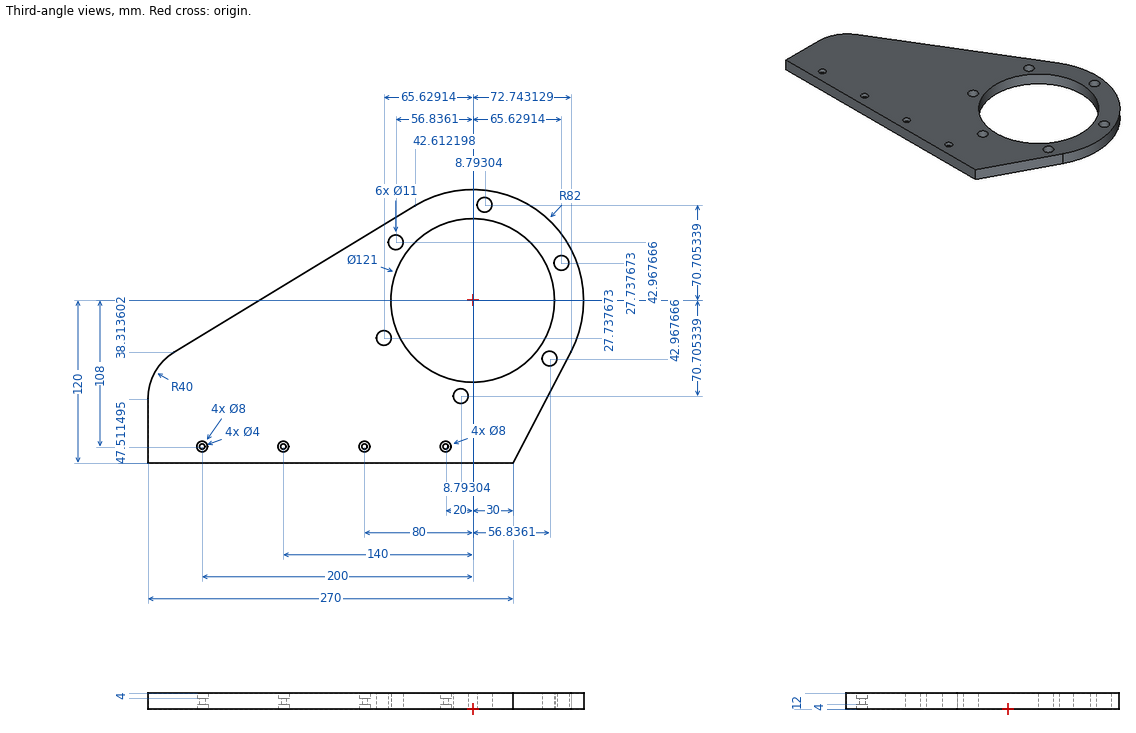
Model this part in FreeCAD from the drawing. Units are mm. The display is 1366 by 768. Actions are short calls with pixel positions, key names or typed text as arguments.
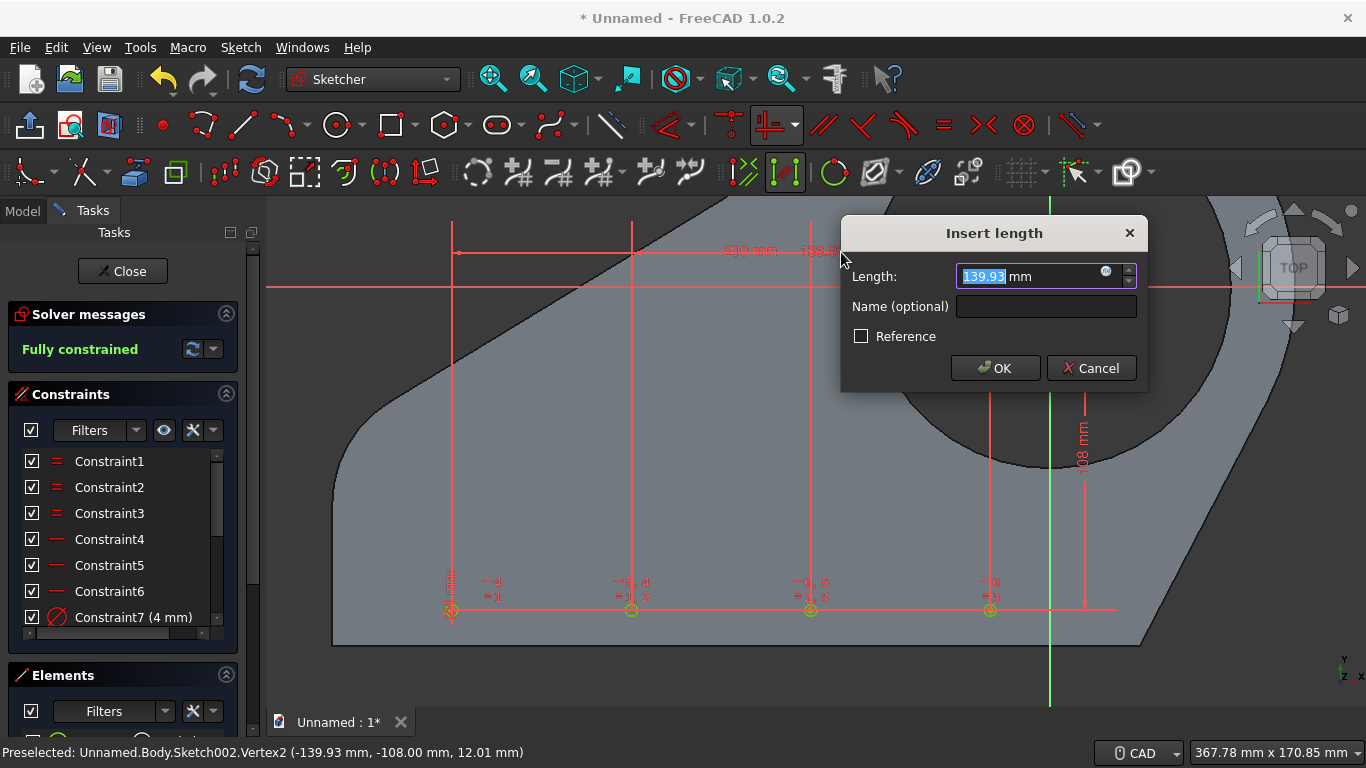
text(140)
key(Return)
key(Escape)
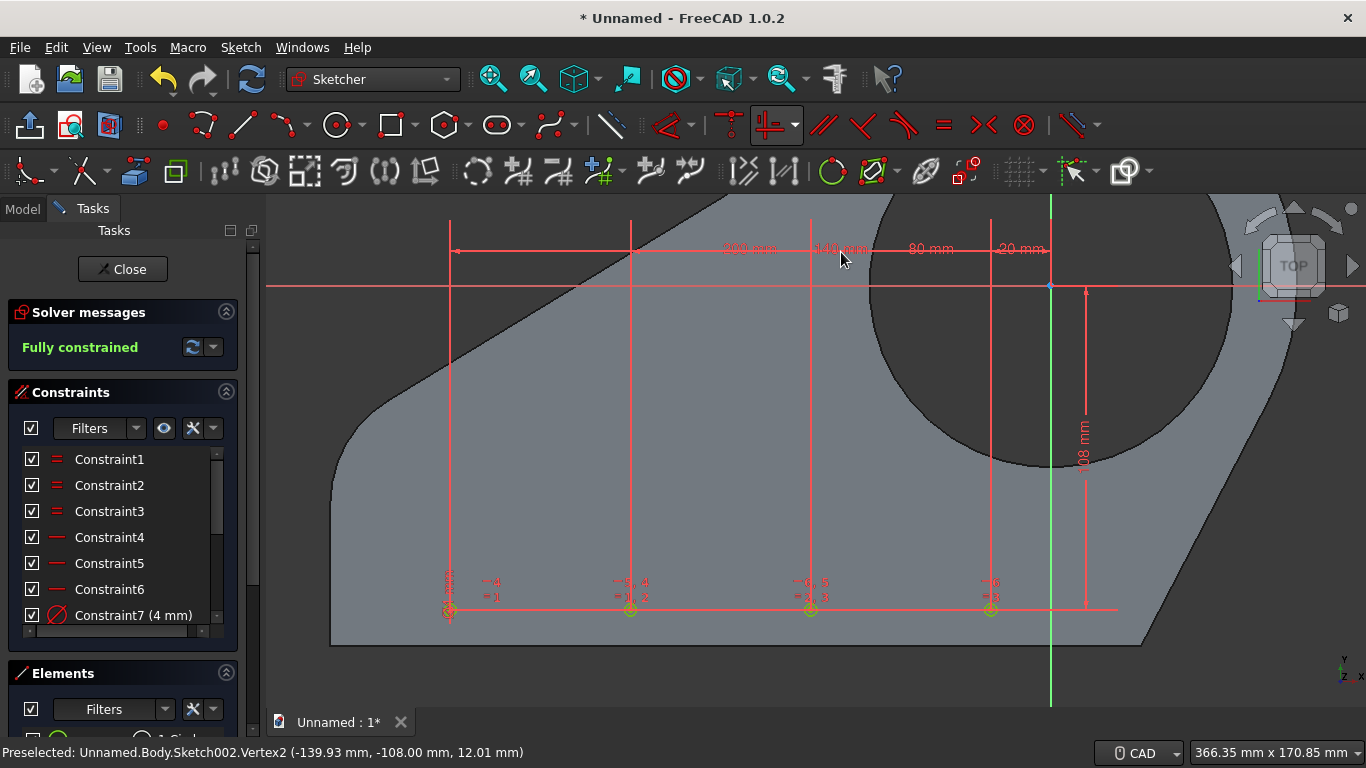
click(123, 269)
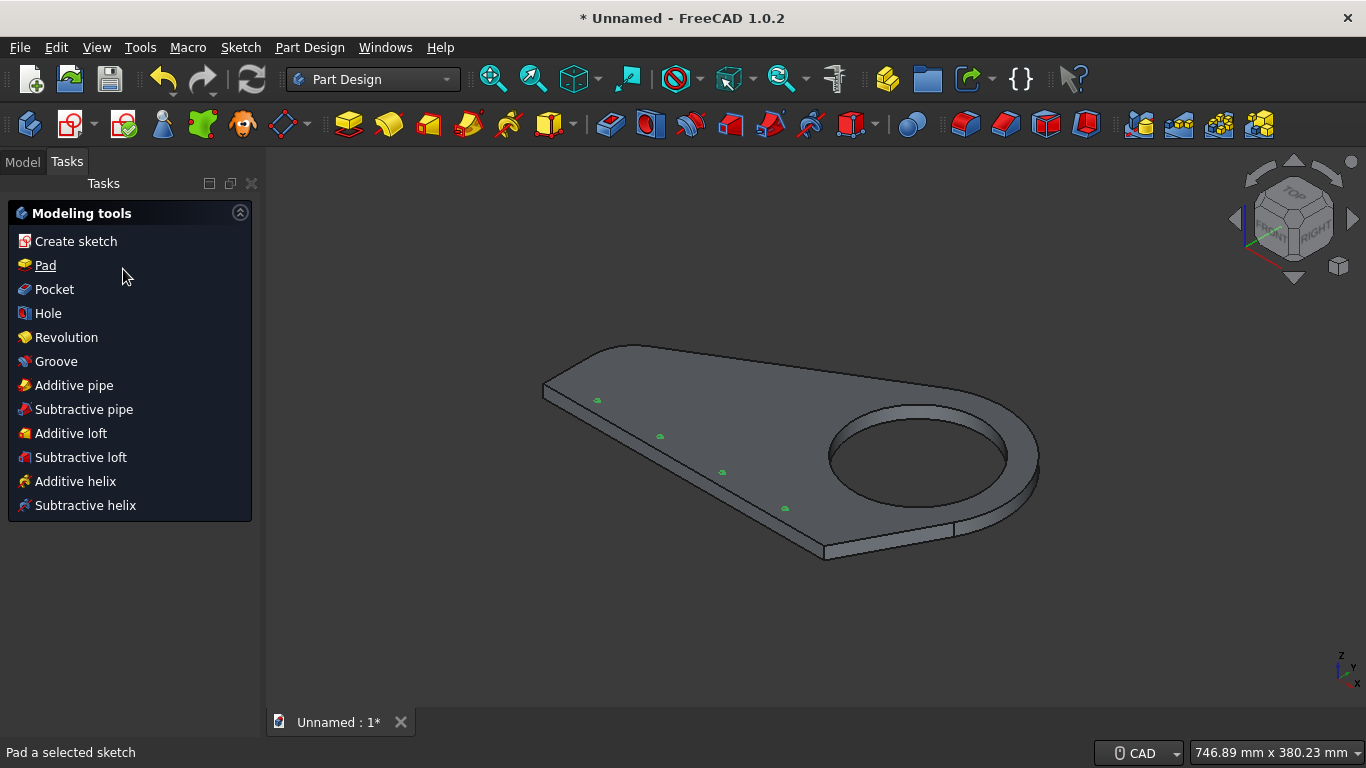
click(612, 124)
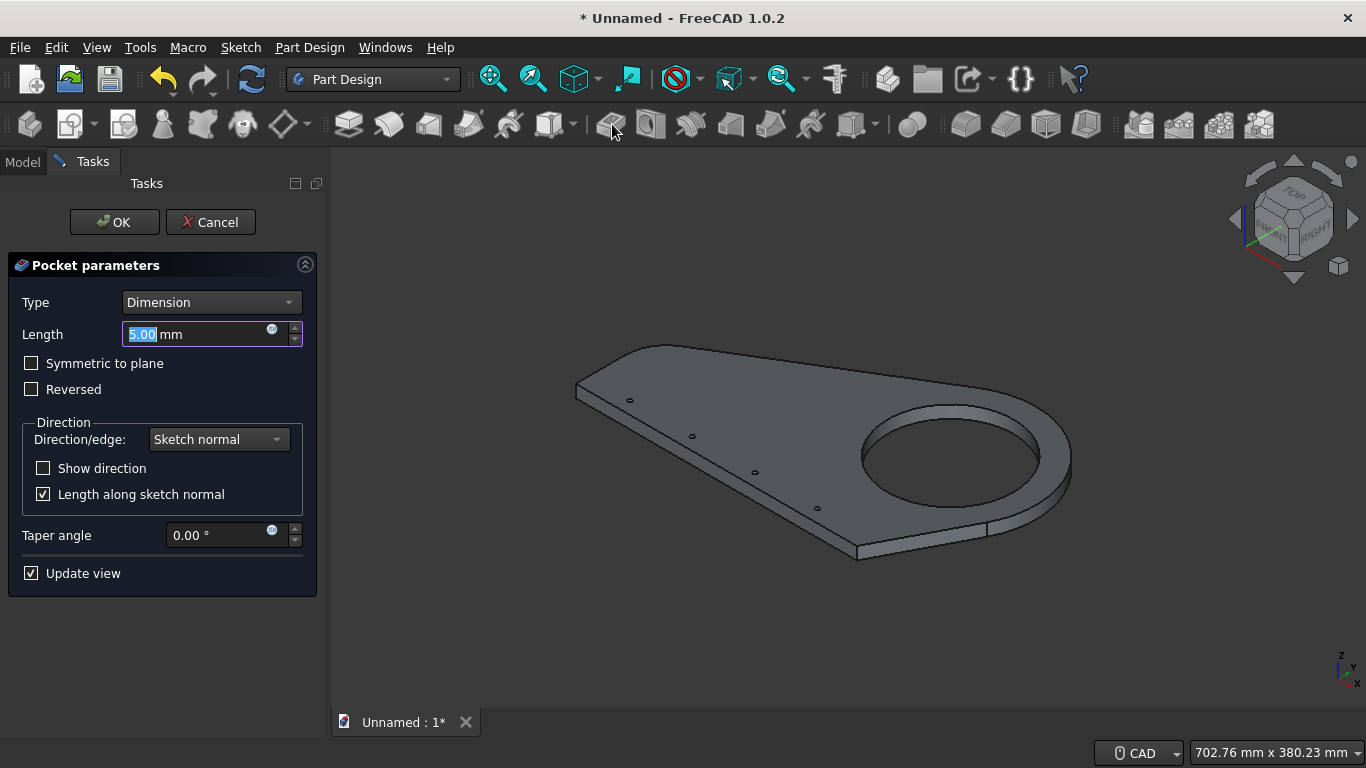
click(212, 302)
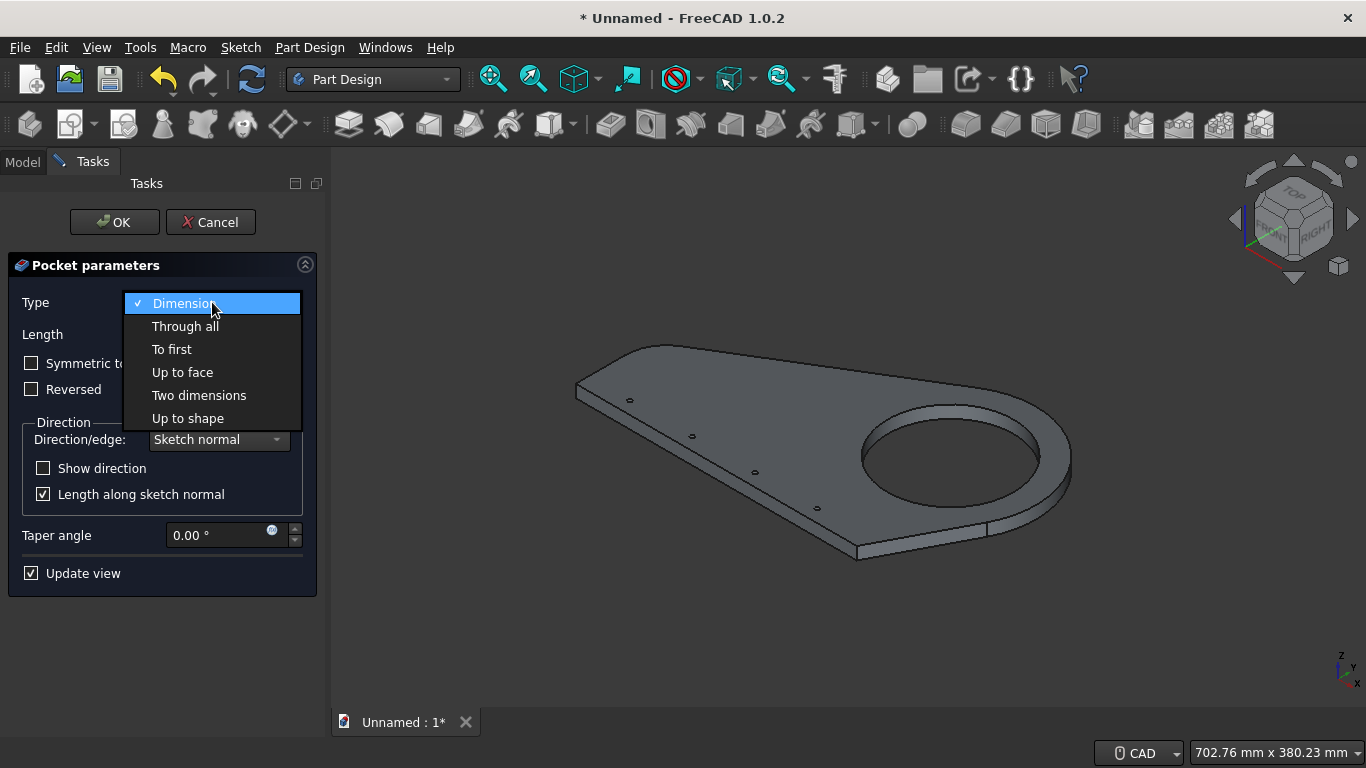
click(212, 326)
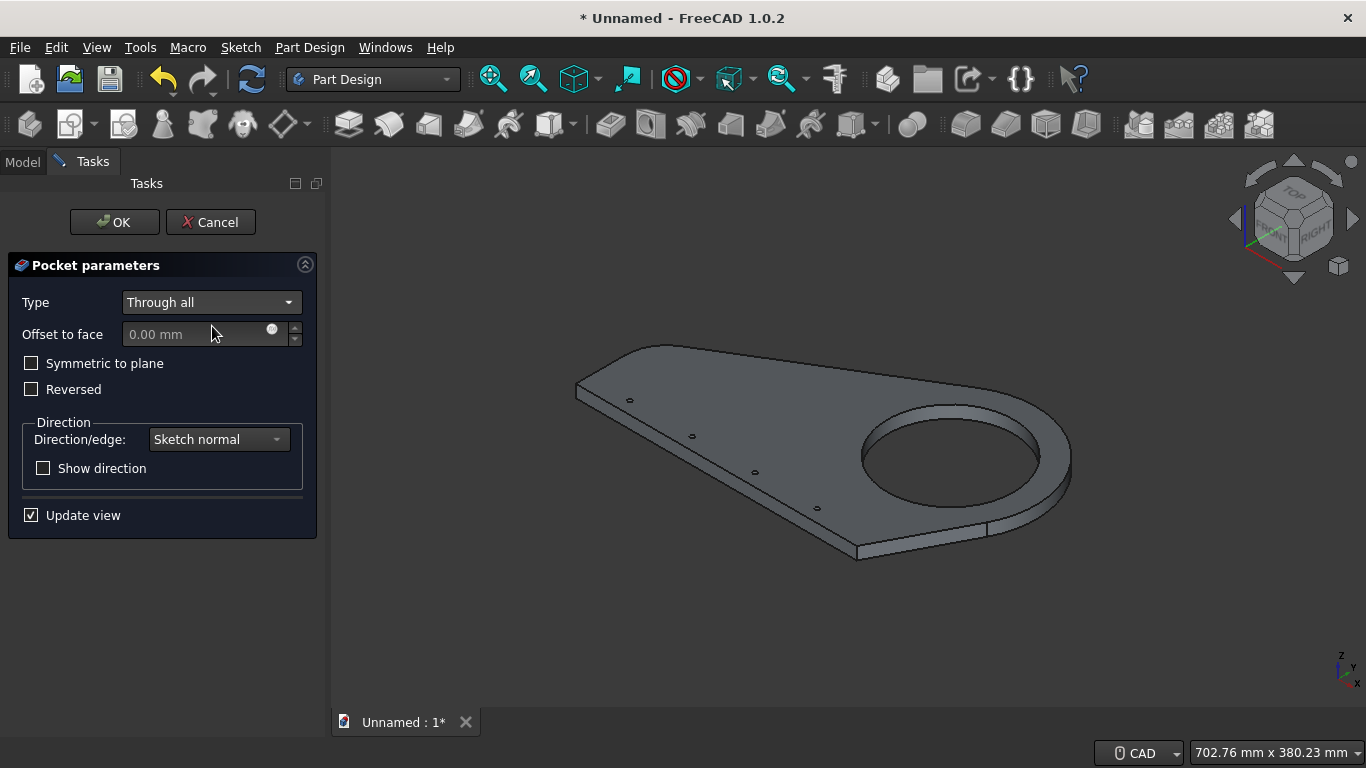
click(115, 222)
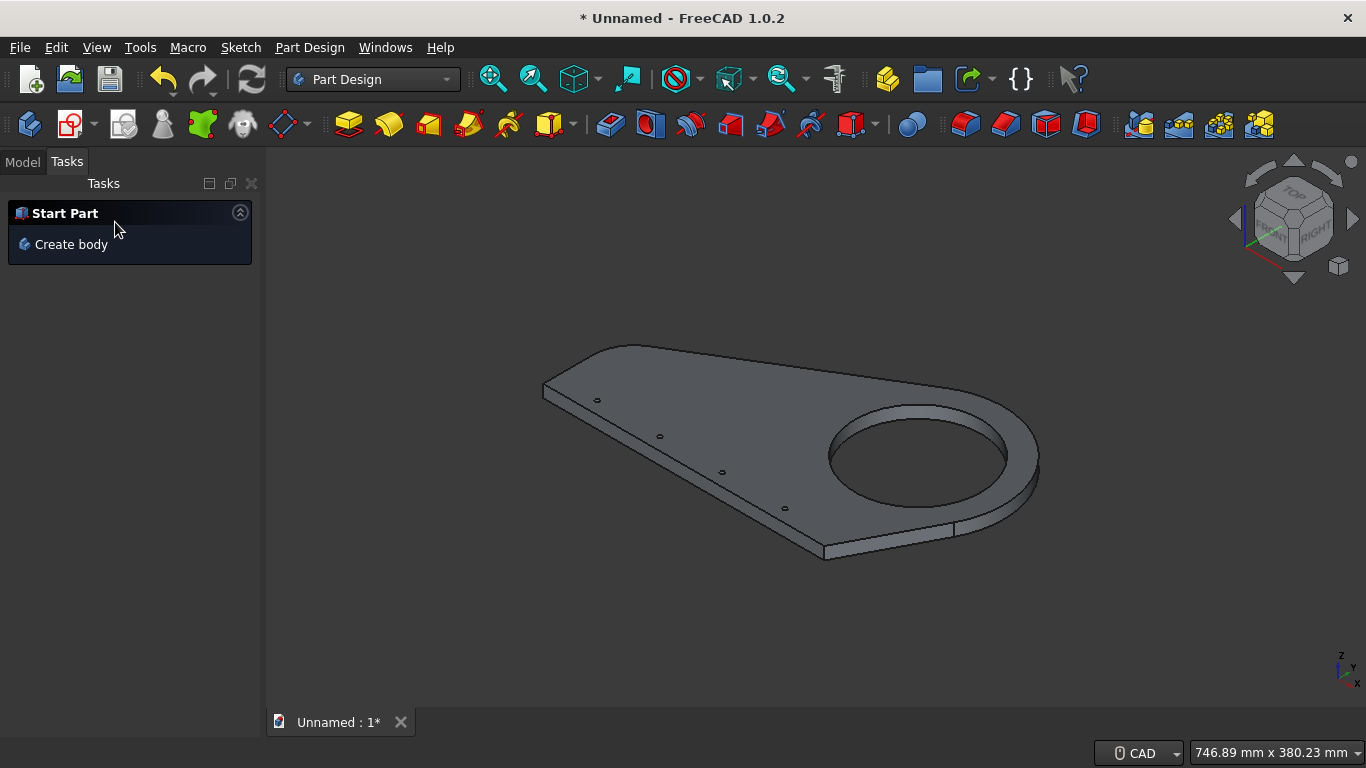
click(738, 408)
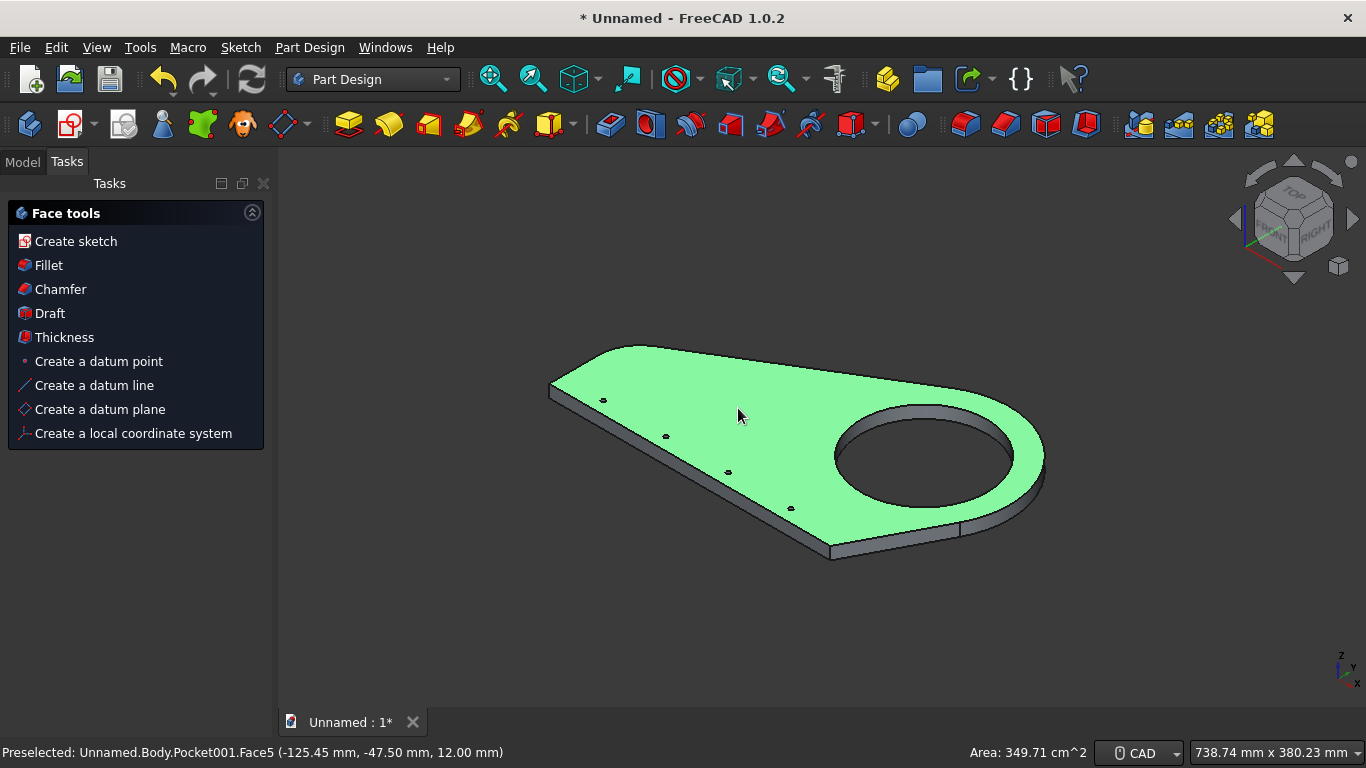
click(70, 124)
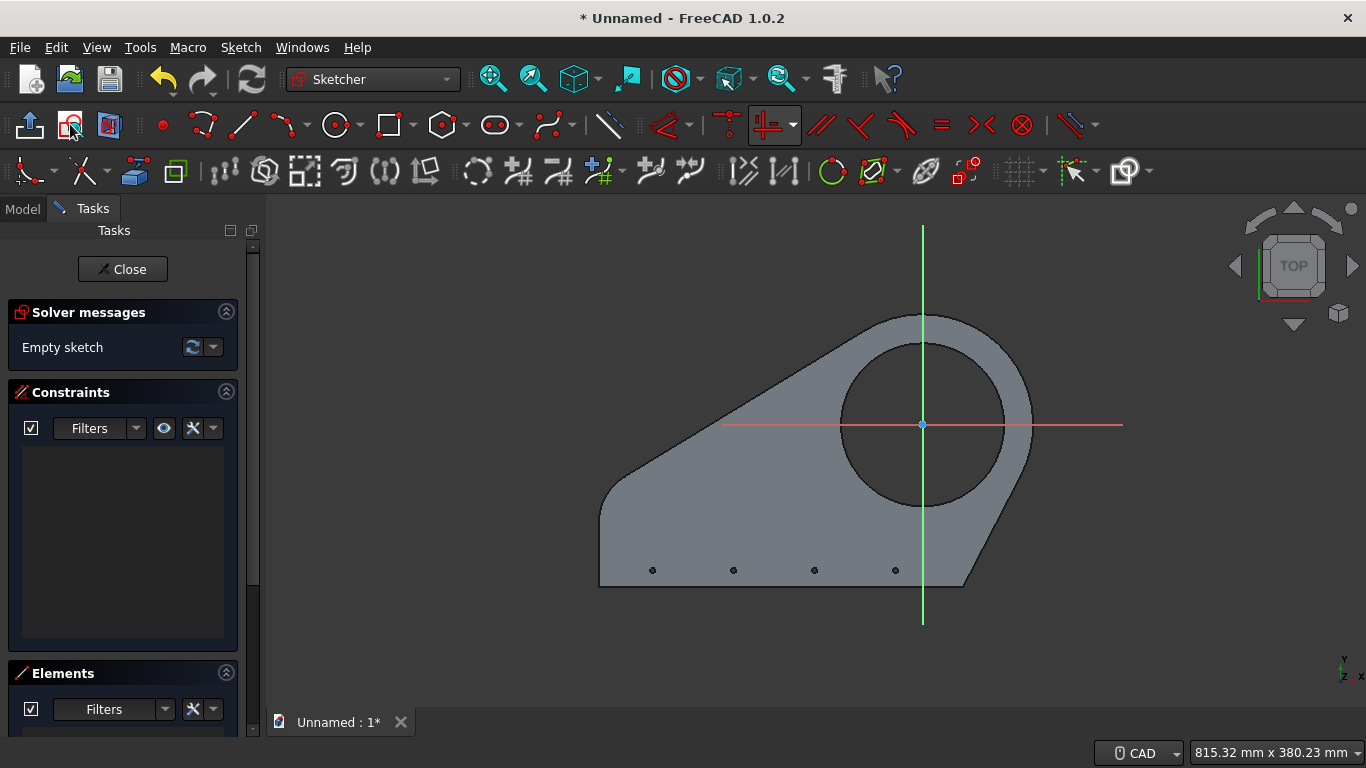
scroll(816, 541, up, 4)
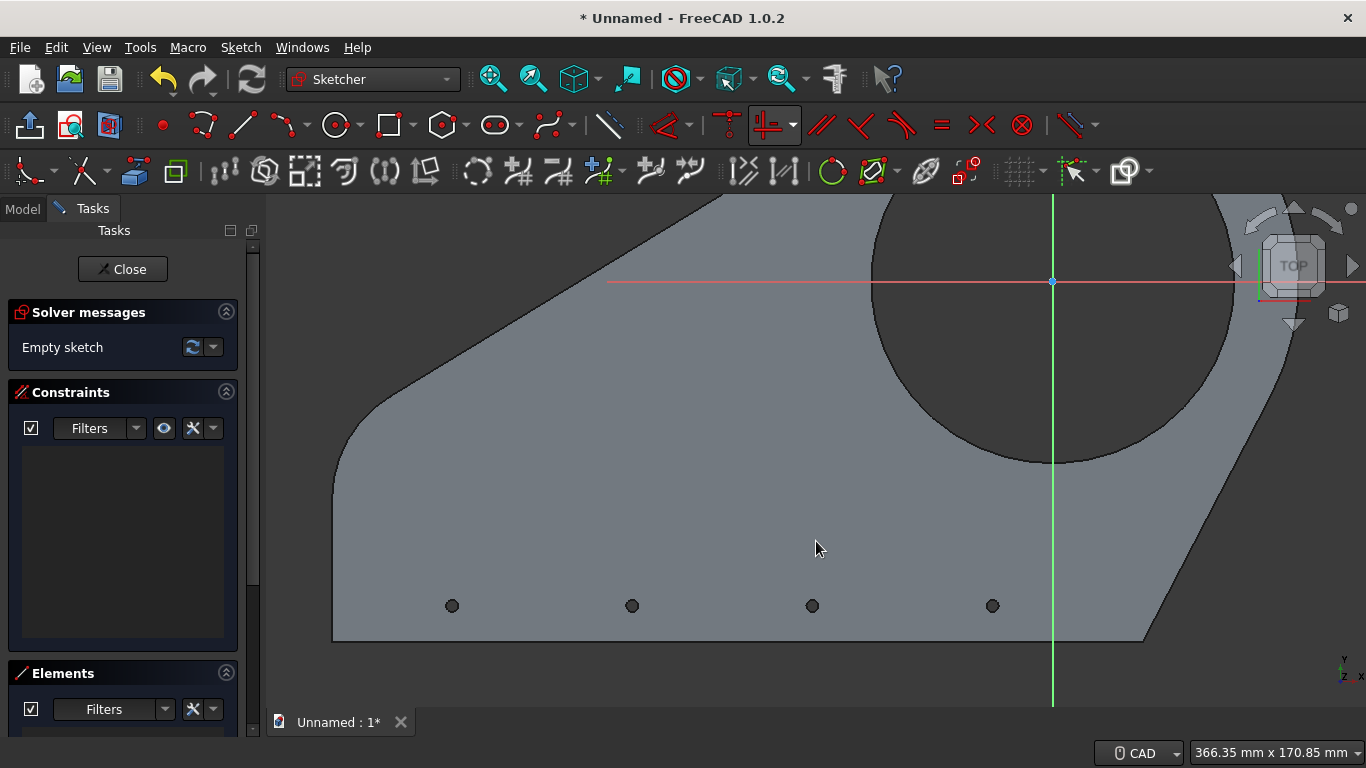
click(336, 126)